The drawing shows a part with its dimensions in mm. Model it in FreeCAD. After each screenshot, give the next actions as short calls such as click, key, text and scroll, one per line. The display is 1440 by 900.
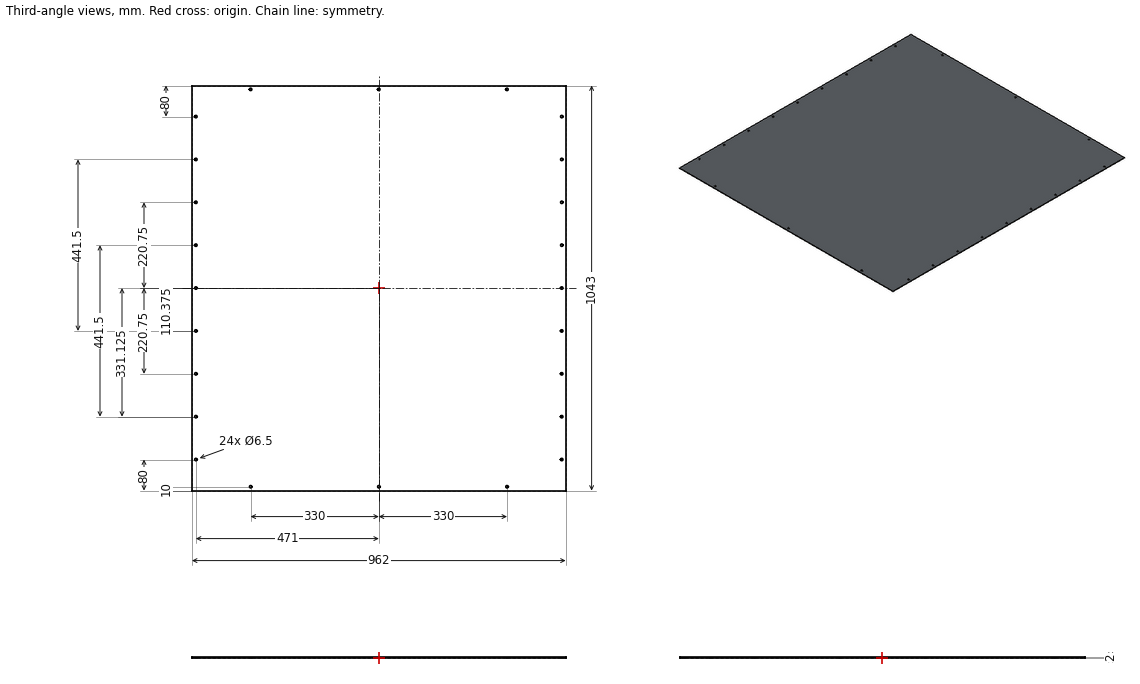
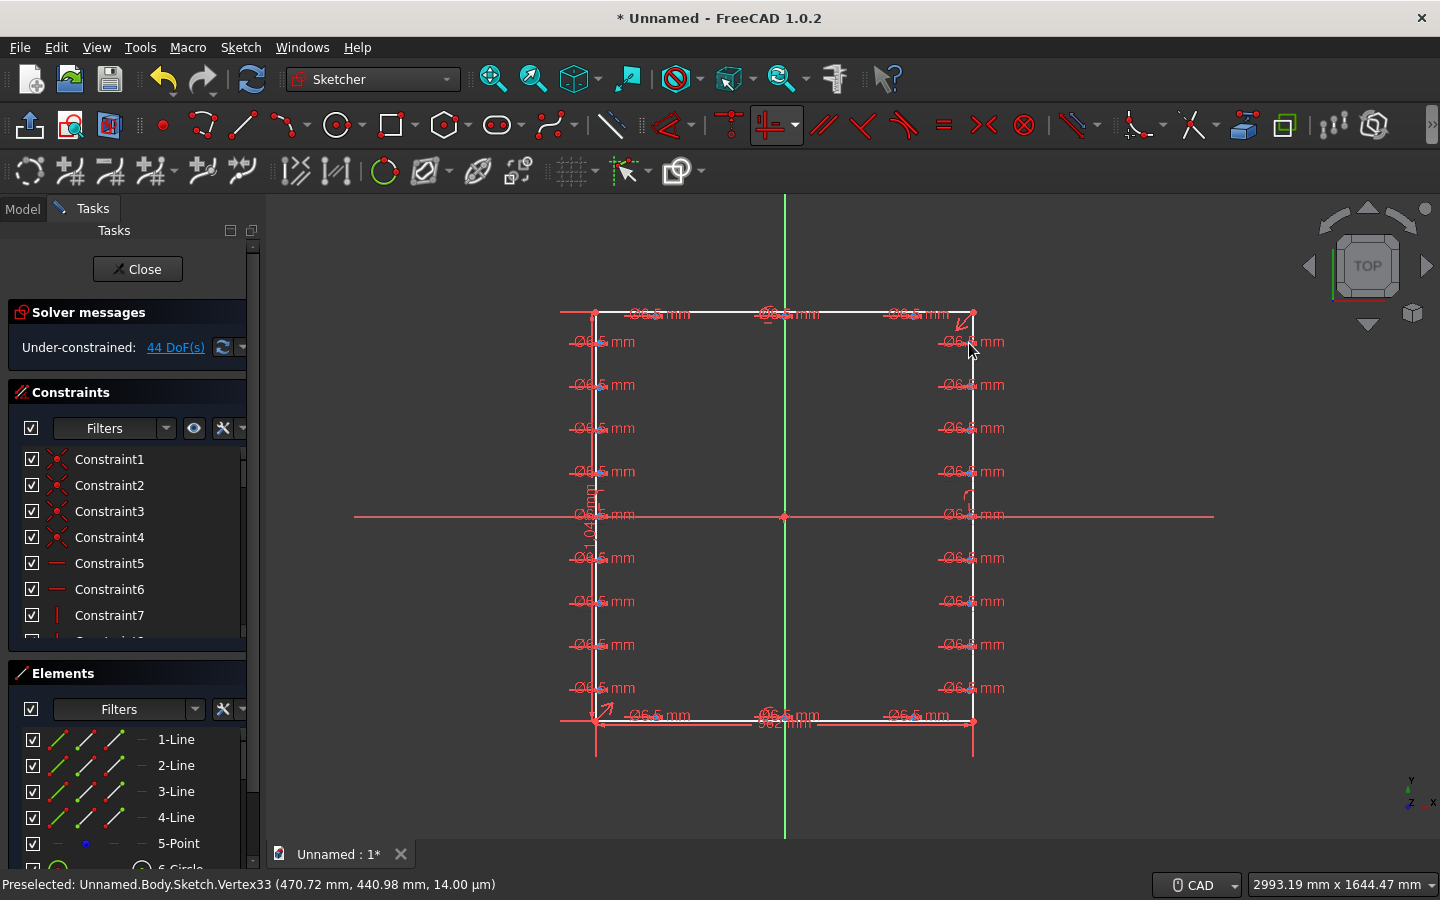
click(600, 690)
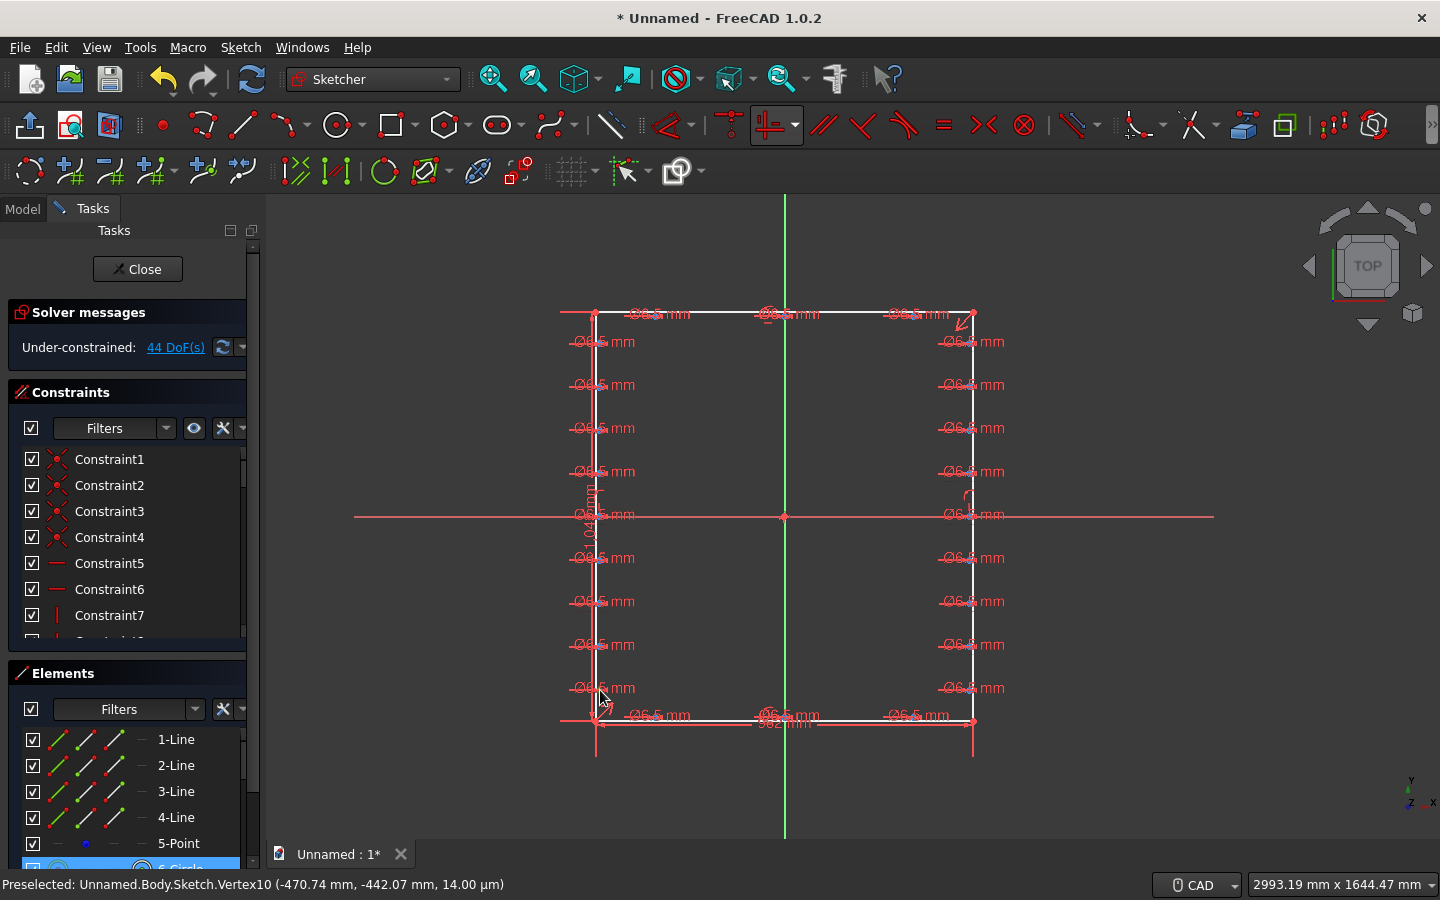
click(600, 647)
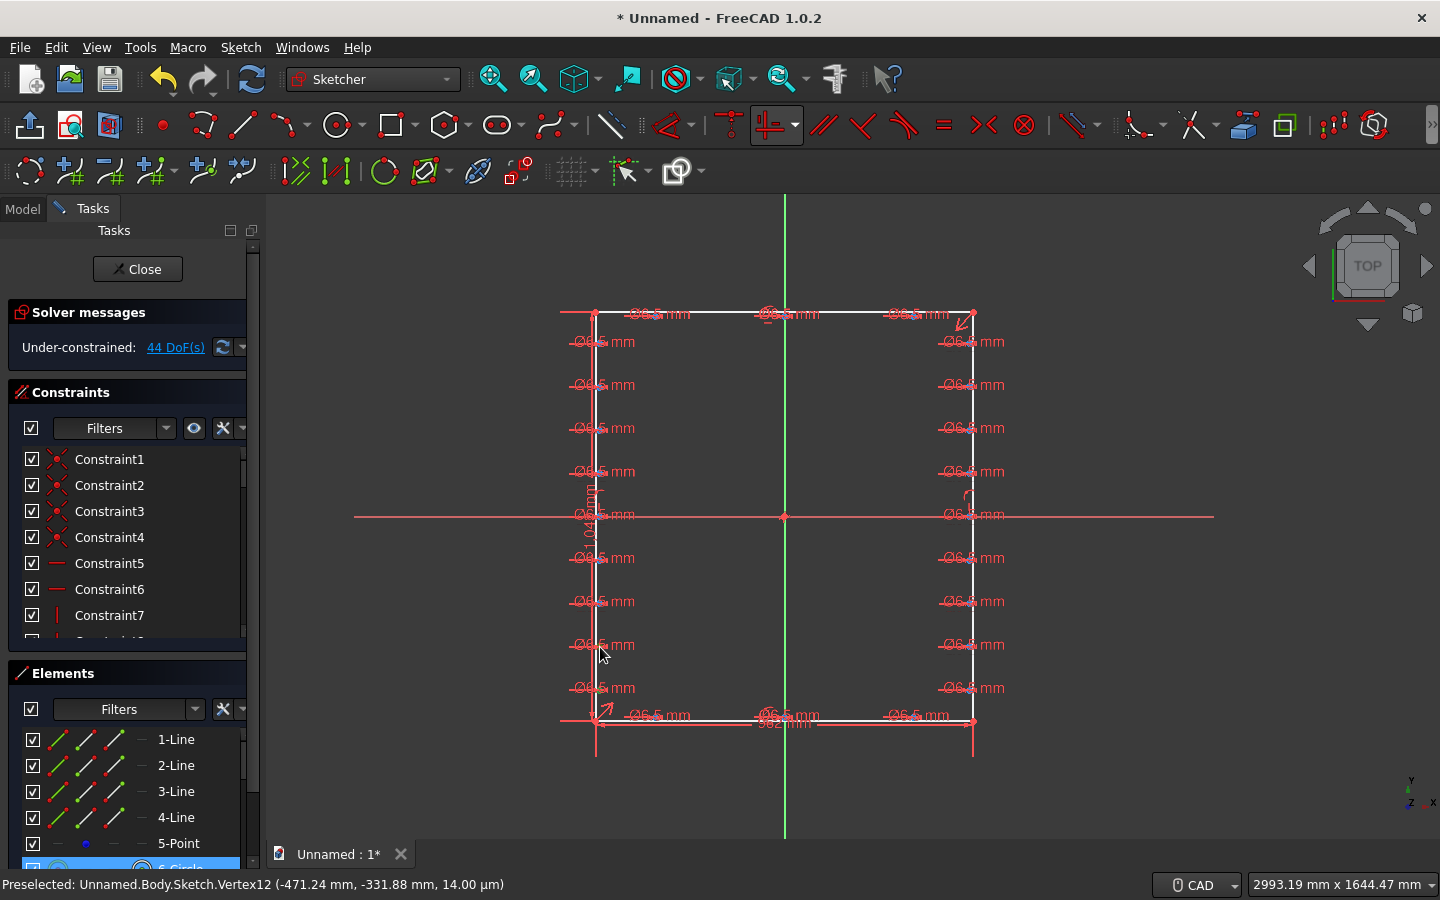
key(v)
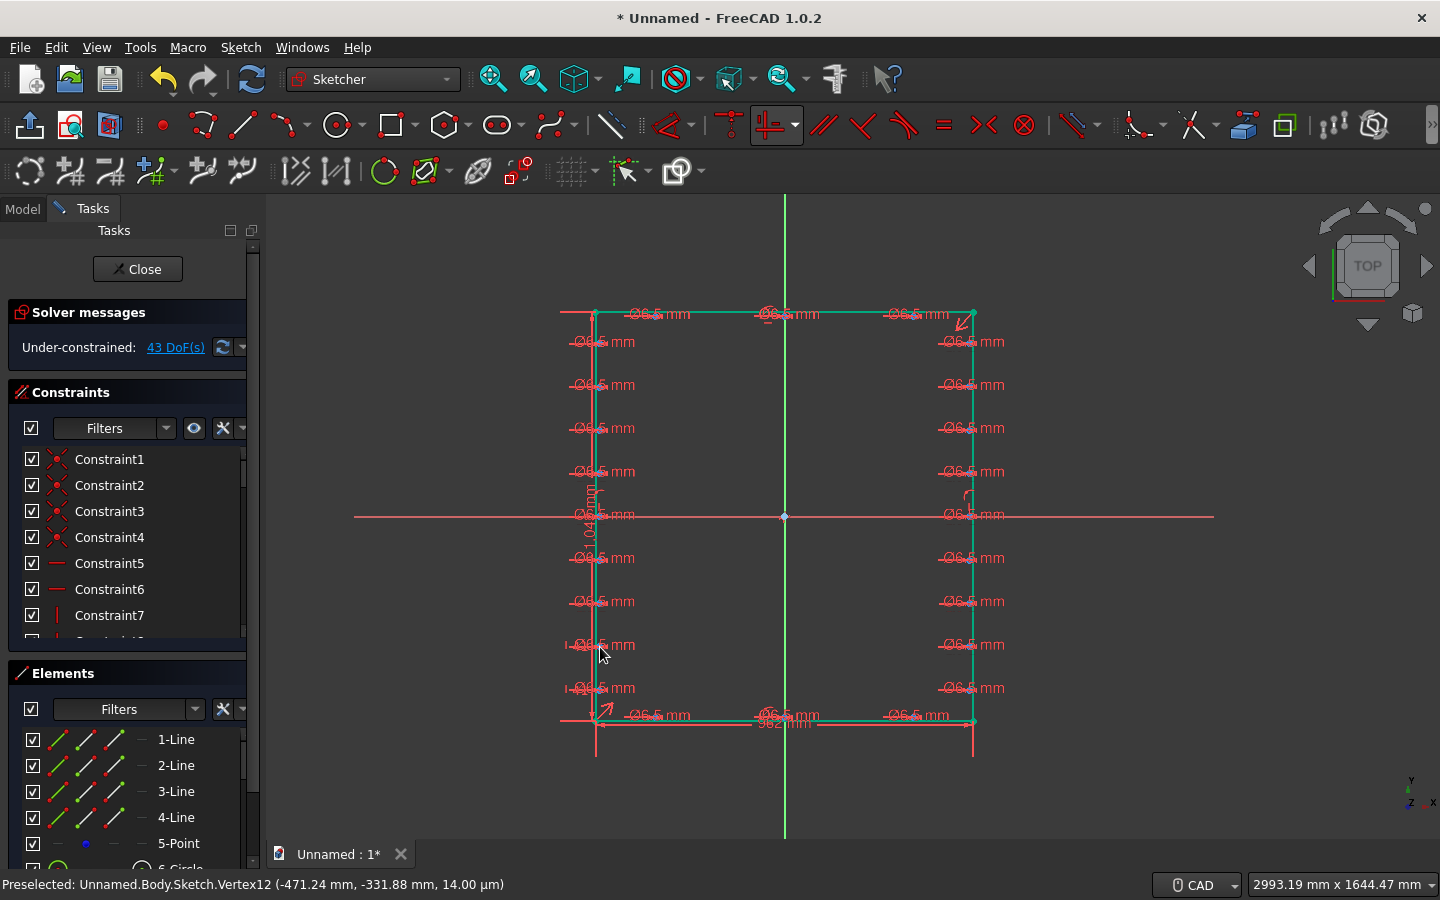
click(600, 647)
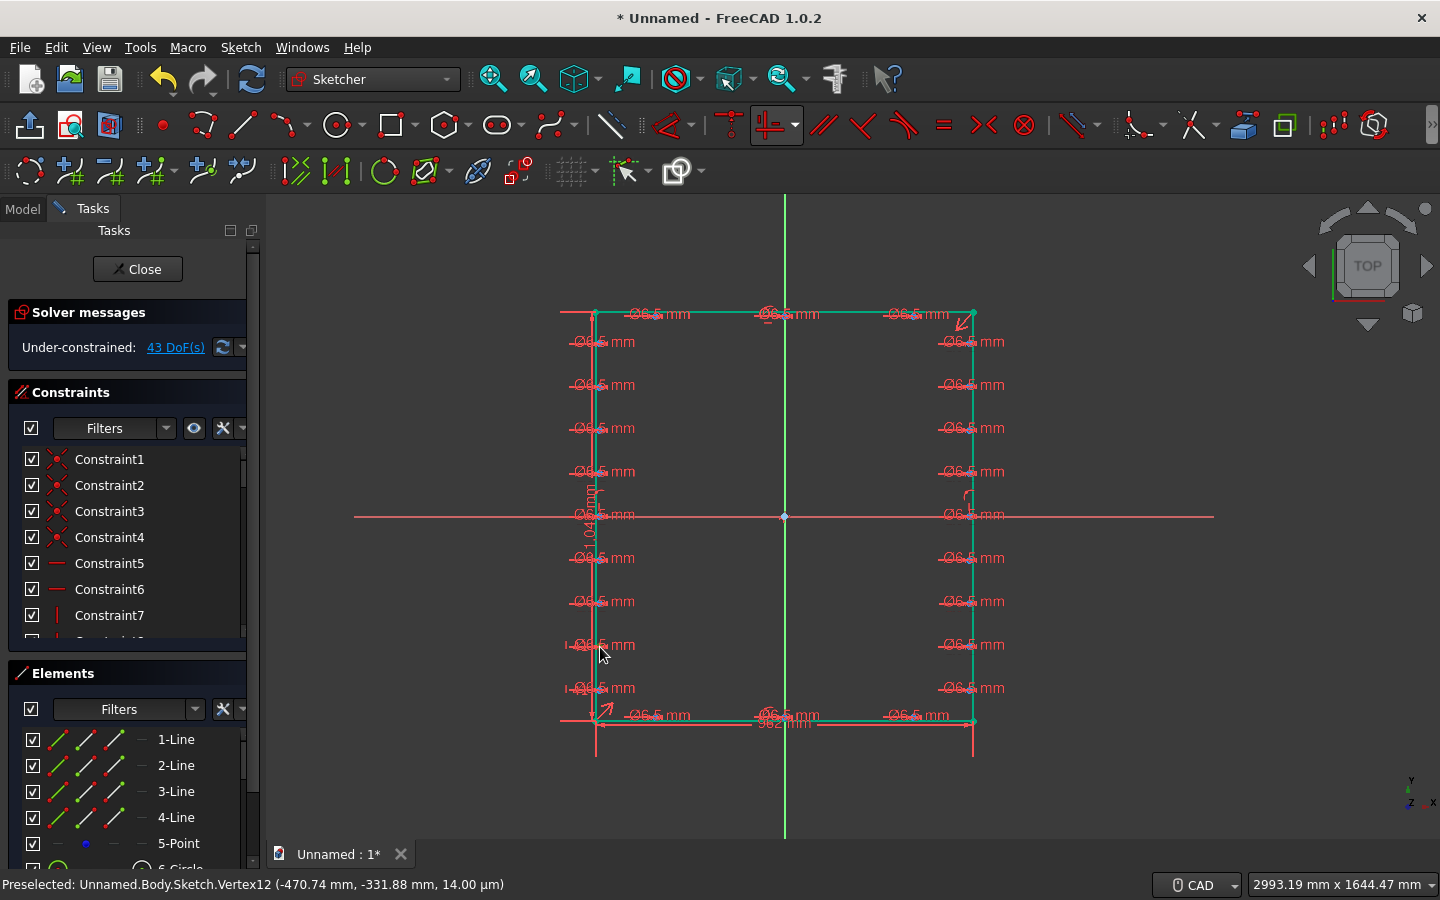
click(600, 604)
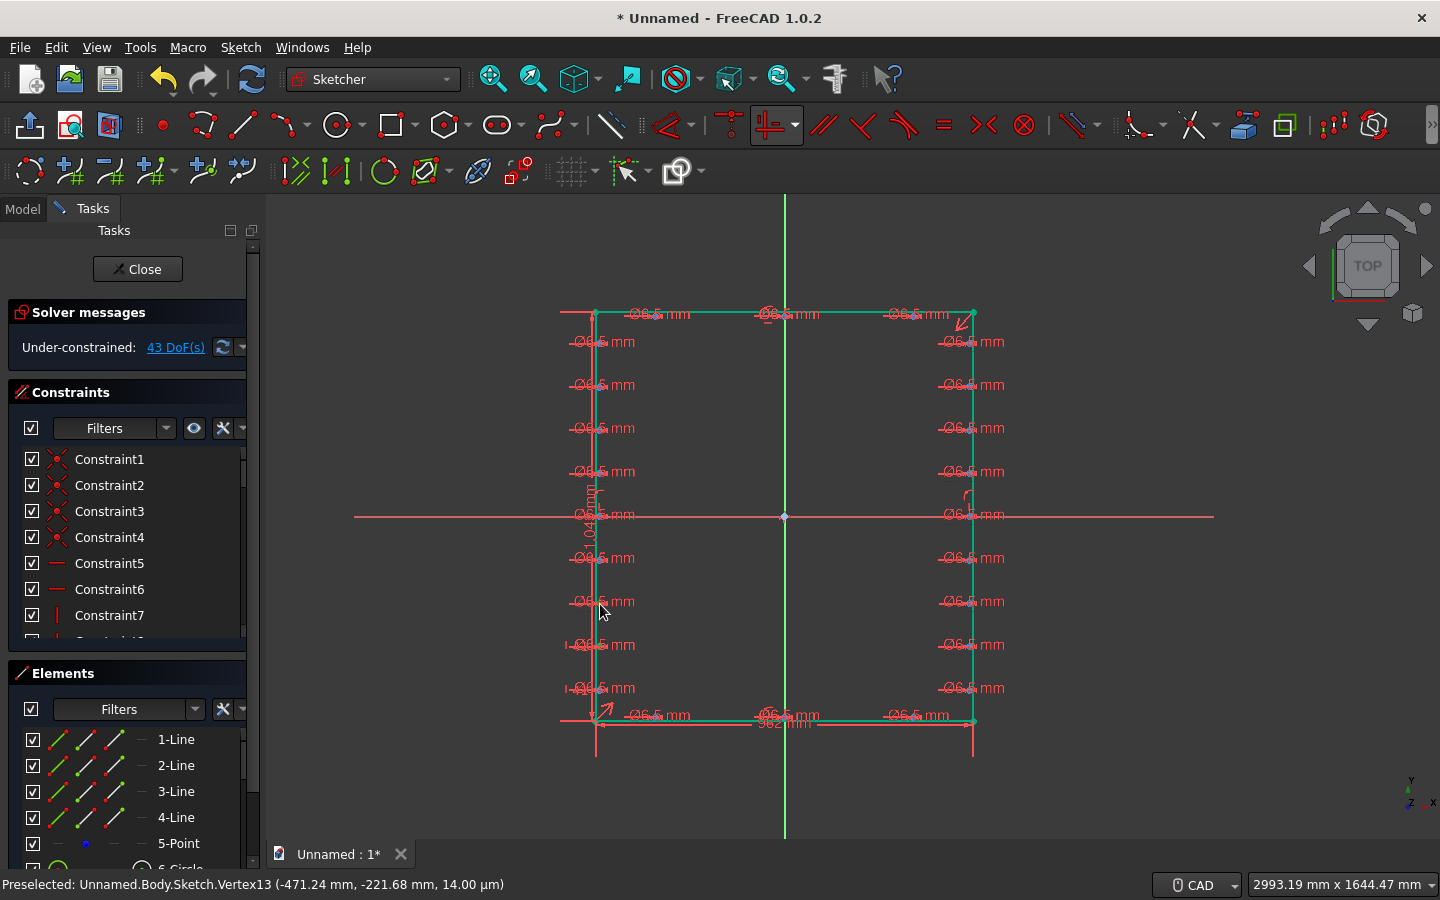
key(v)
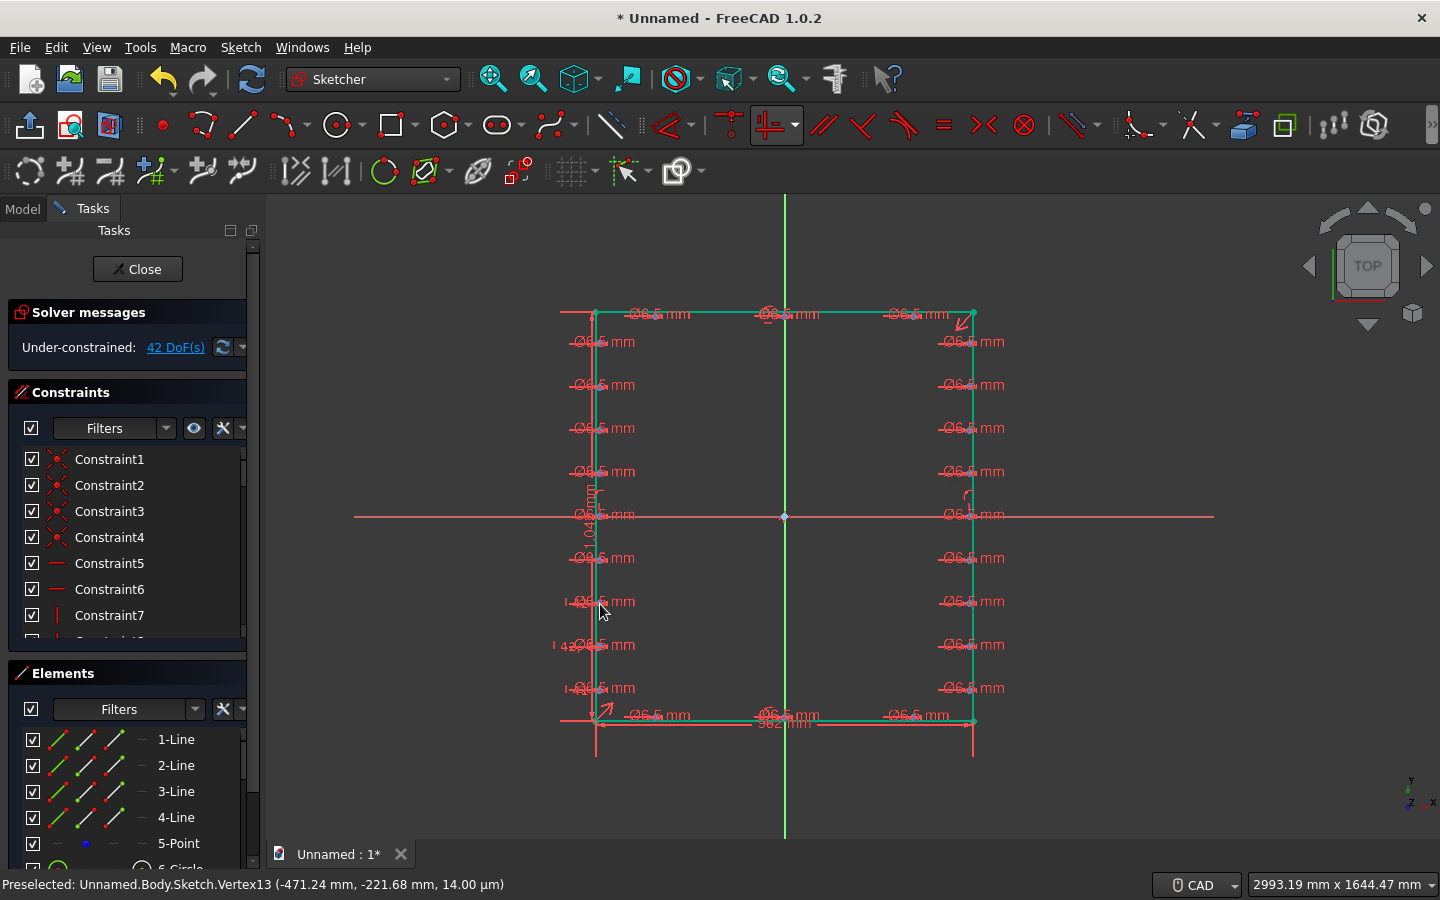
click(600, 604)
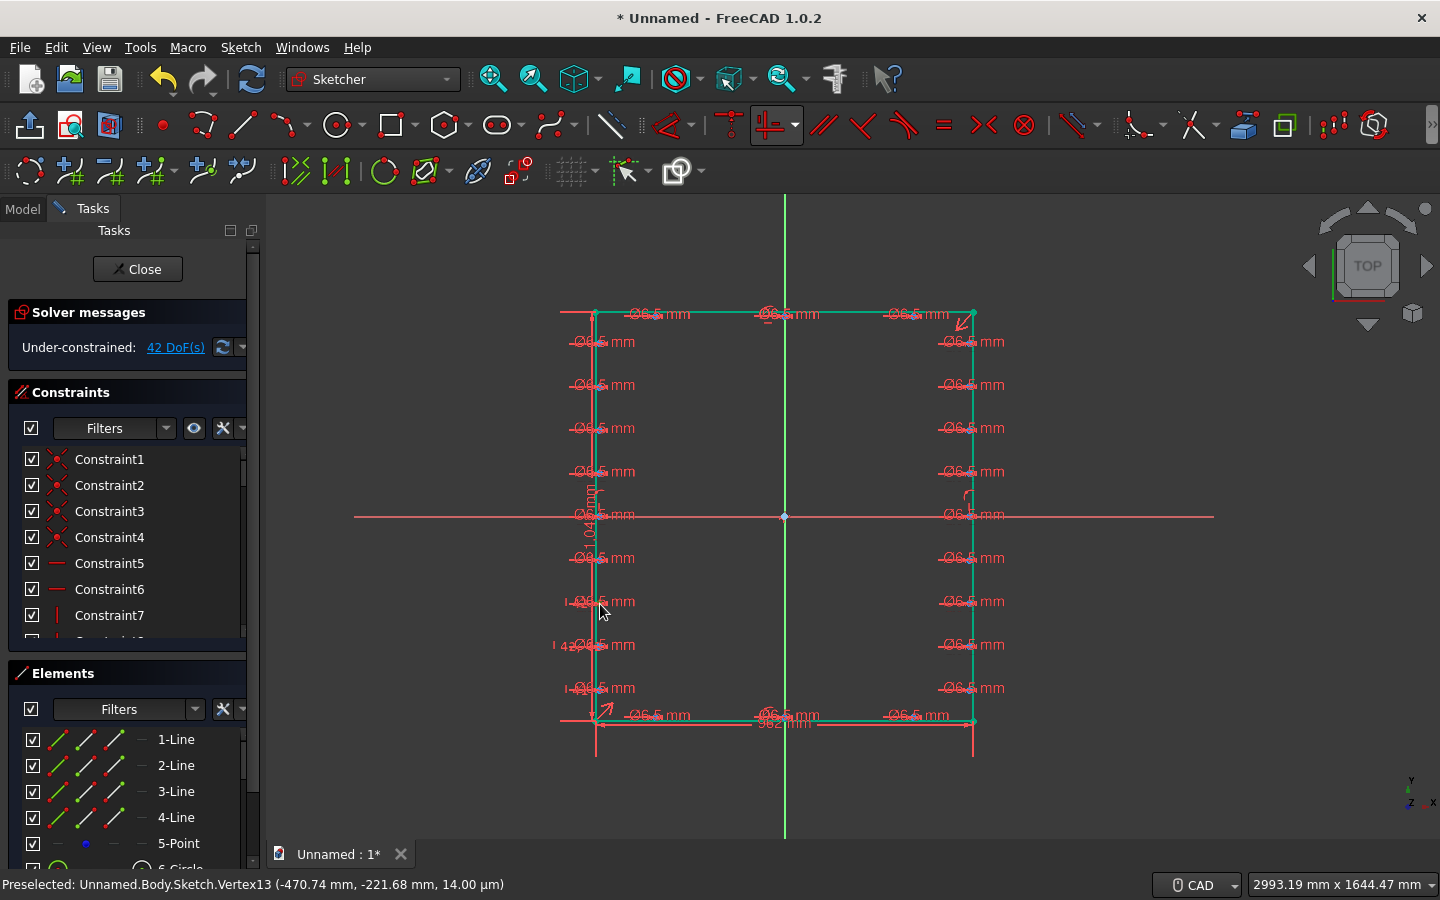
click(600, 560)